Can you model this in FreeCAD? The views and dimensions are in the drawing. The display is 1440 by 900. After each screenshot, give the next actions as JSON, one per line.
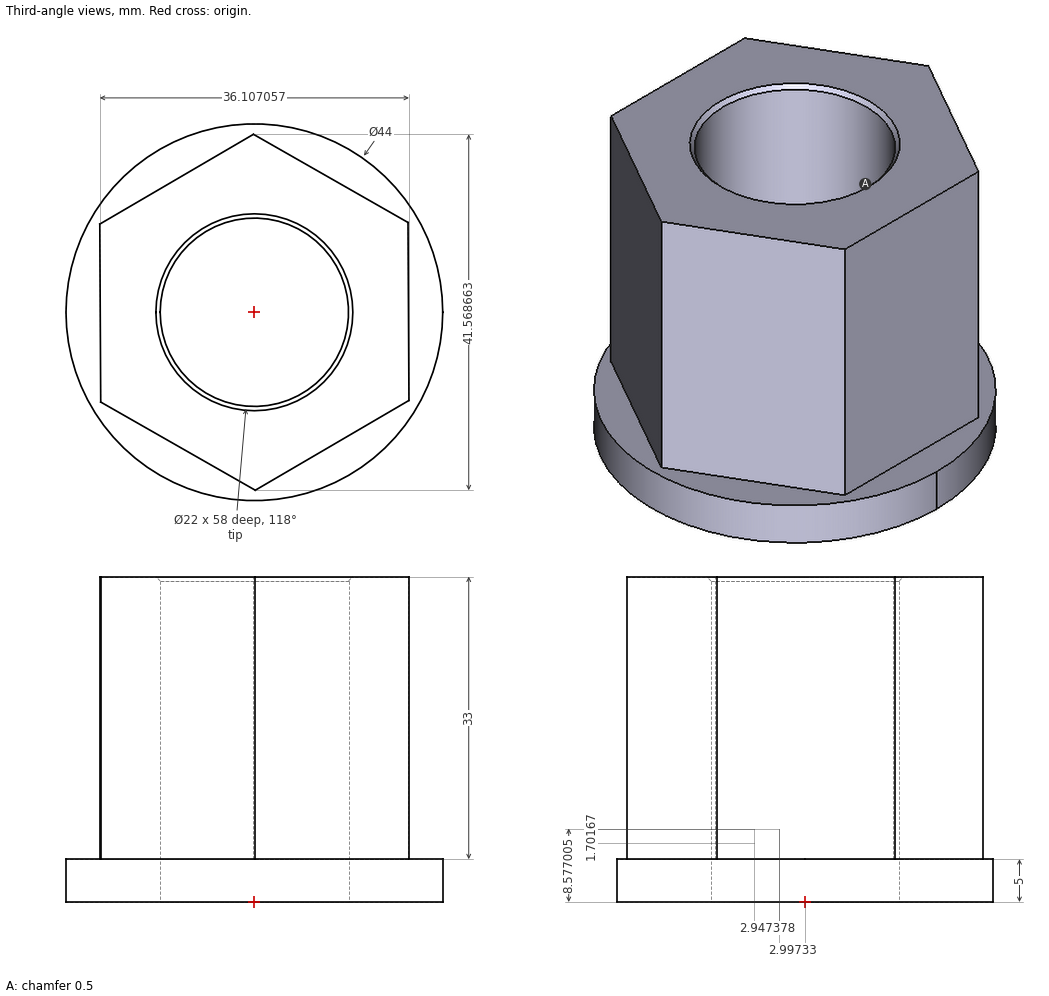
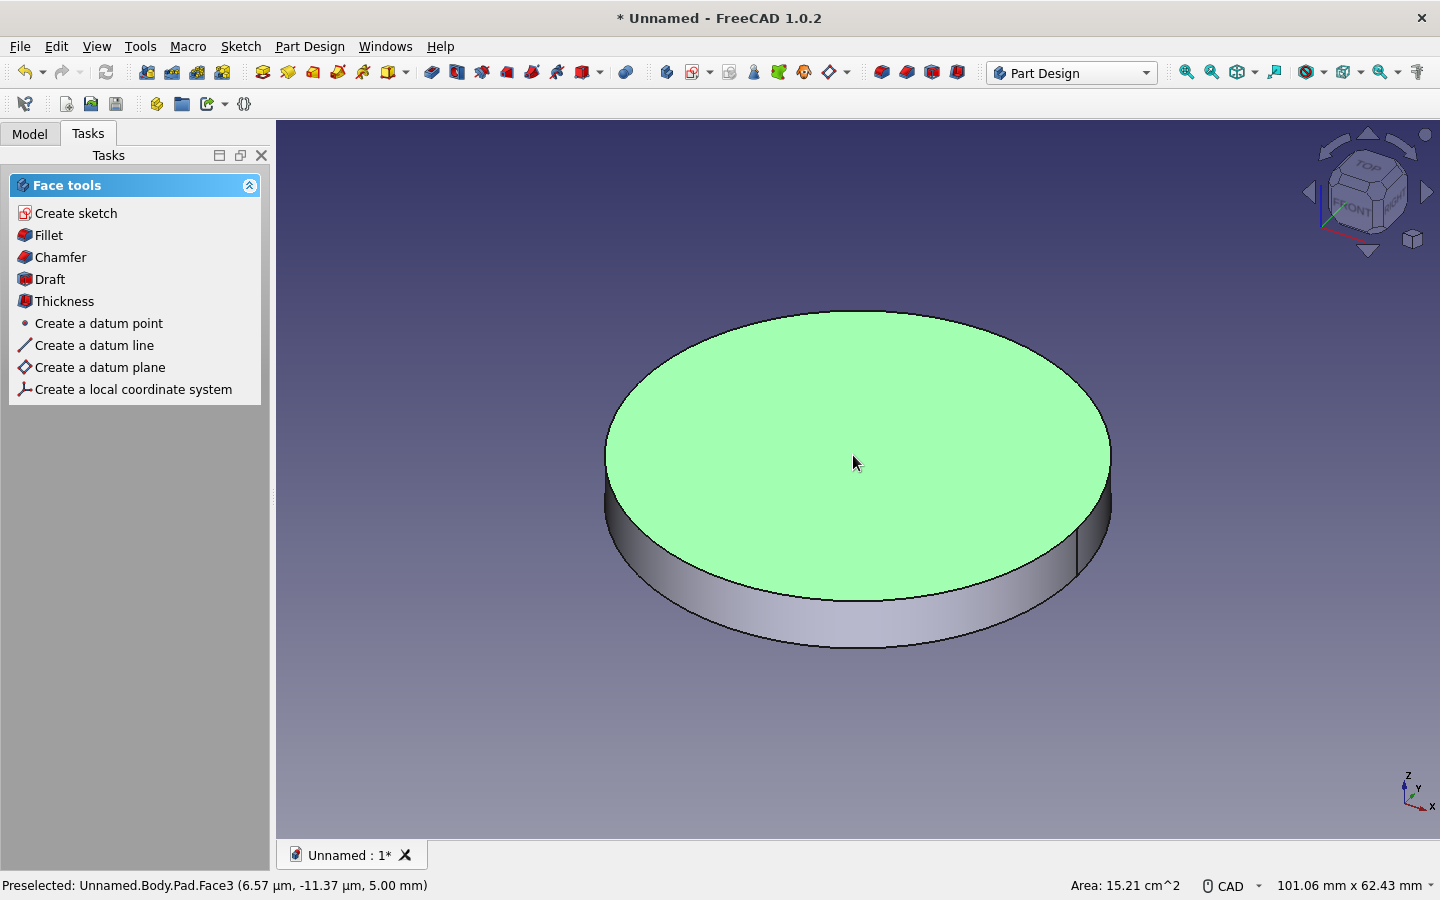
{"action": "left_click", "coordinate": [692, 72]}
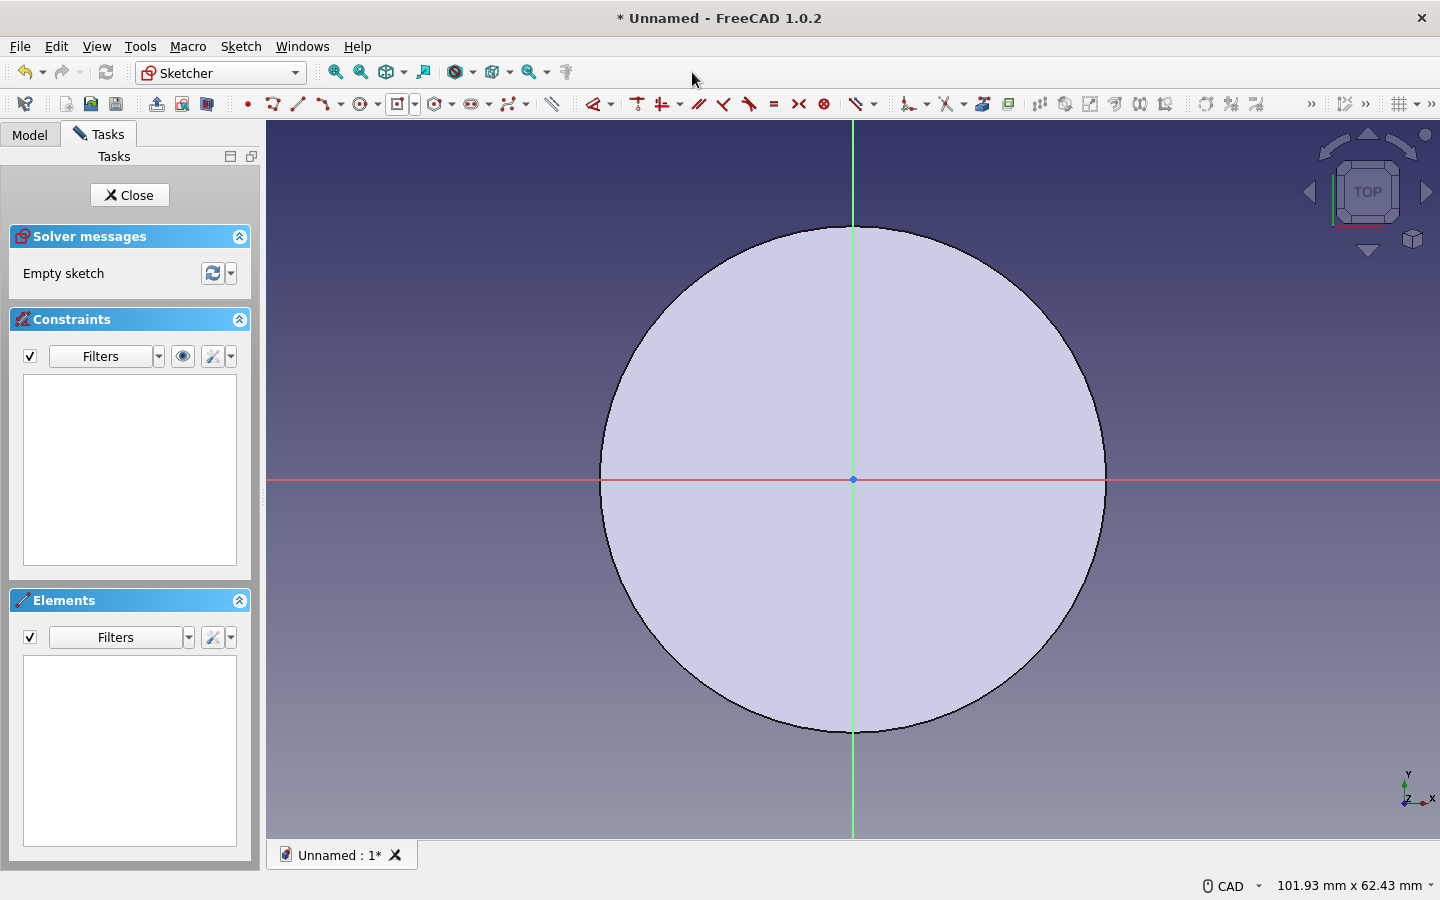
{"action": "key", "text": "g p 6"}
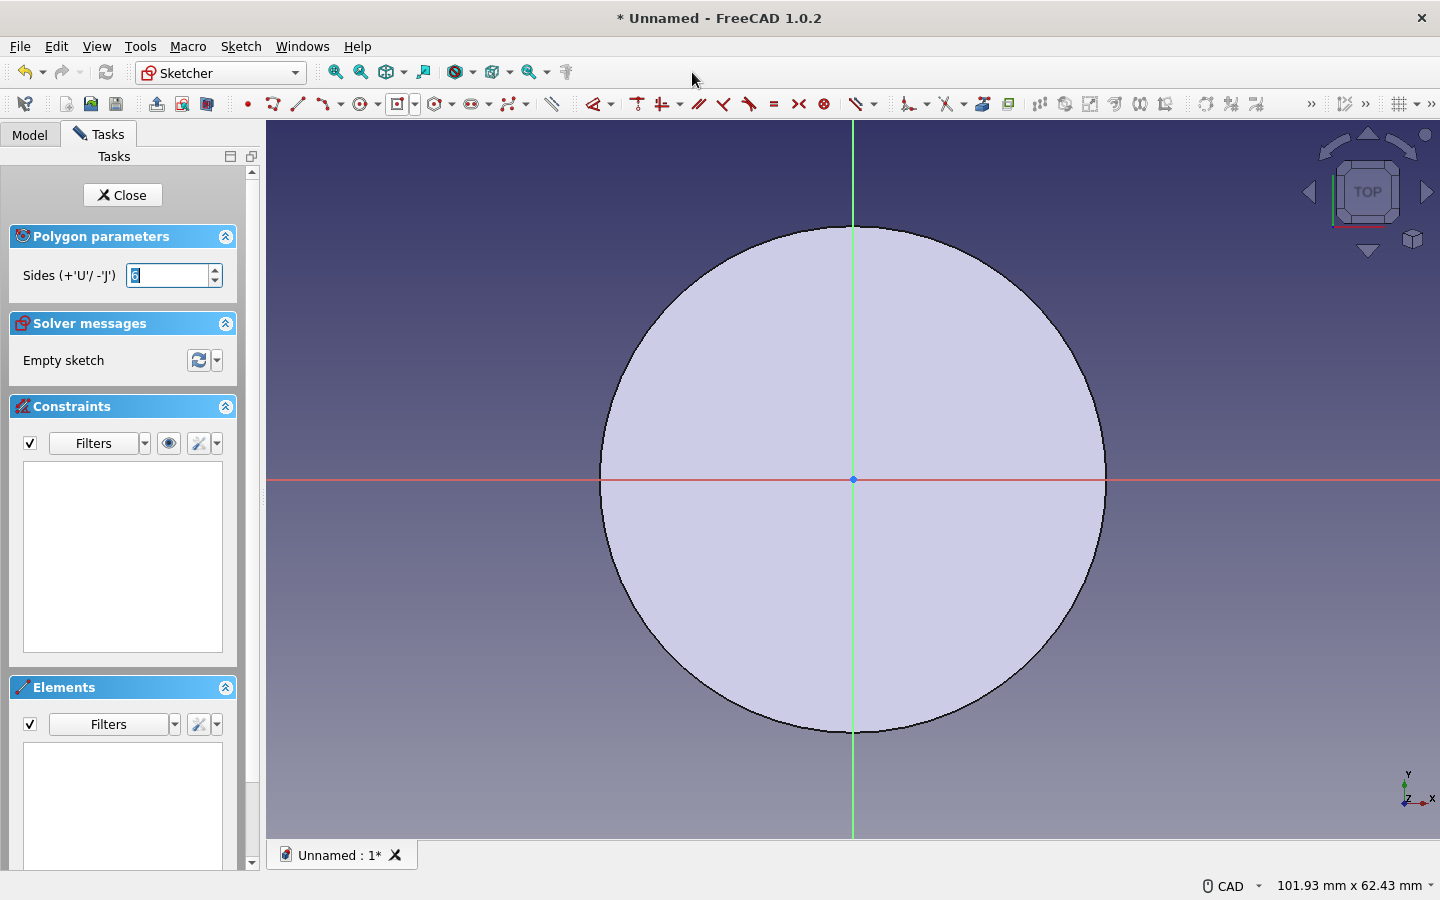
{"action": "left_click", "coordinate": [853, 480]}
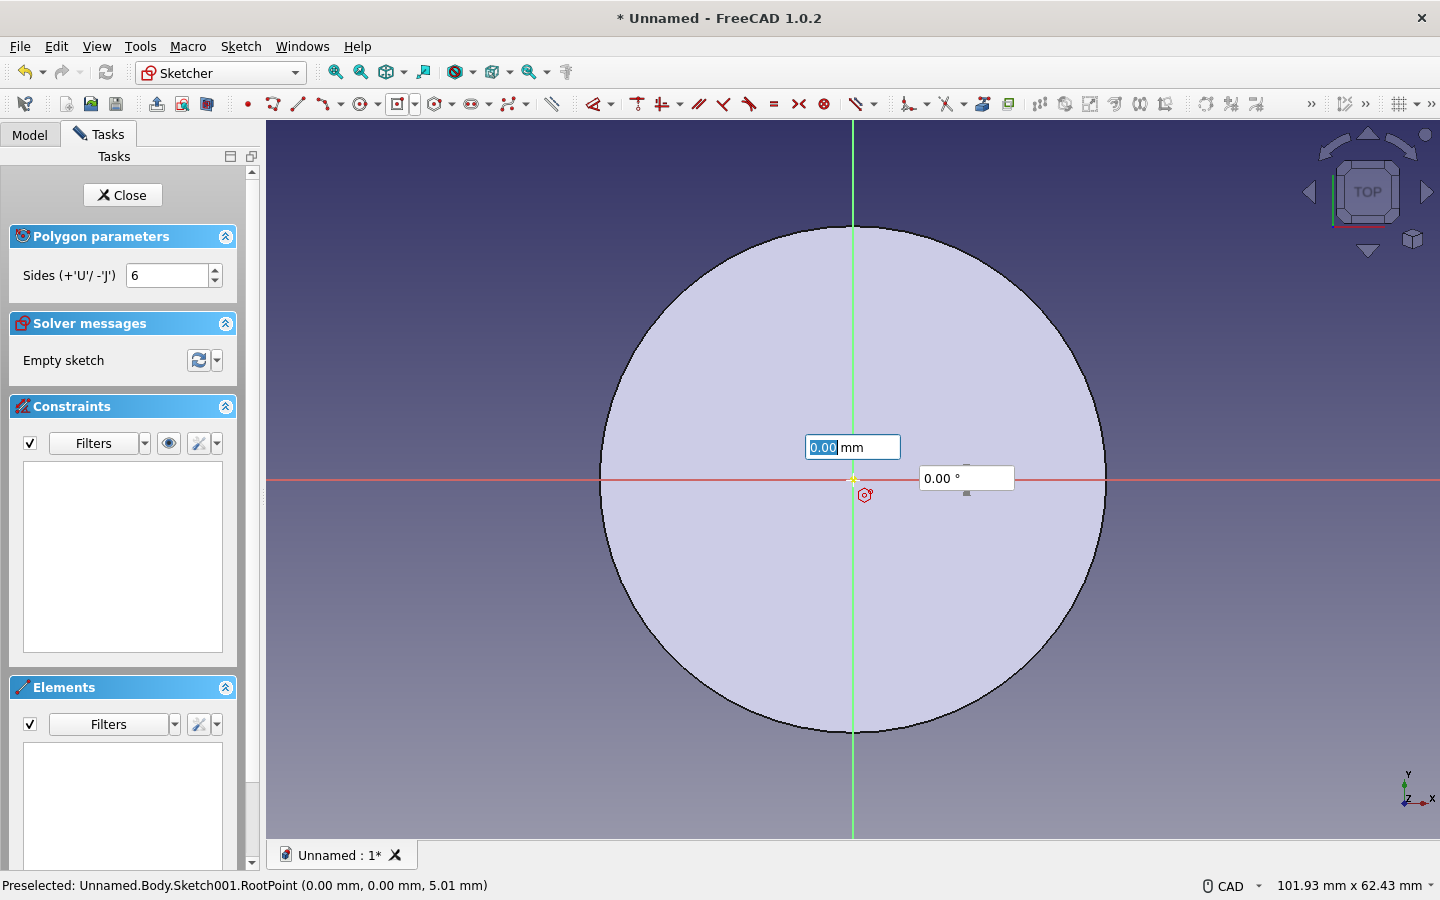
{"action": "left_click", "coordinate": [646, 600]}
{"action": "right_click", "coordinate": [646, 600]}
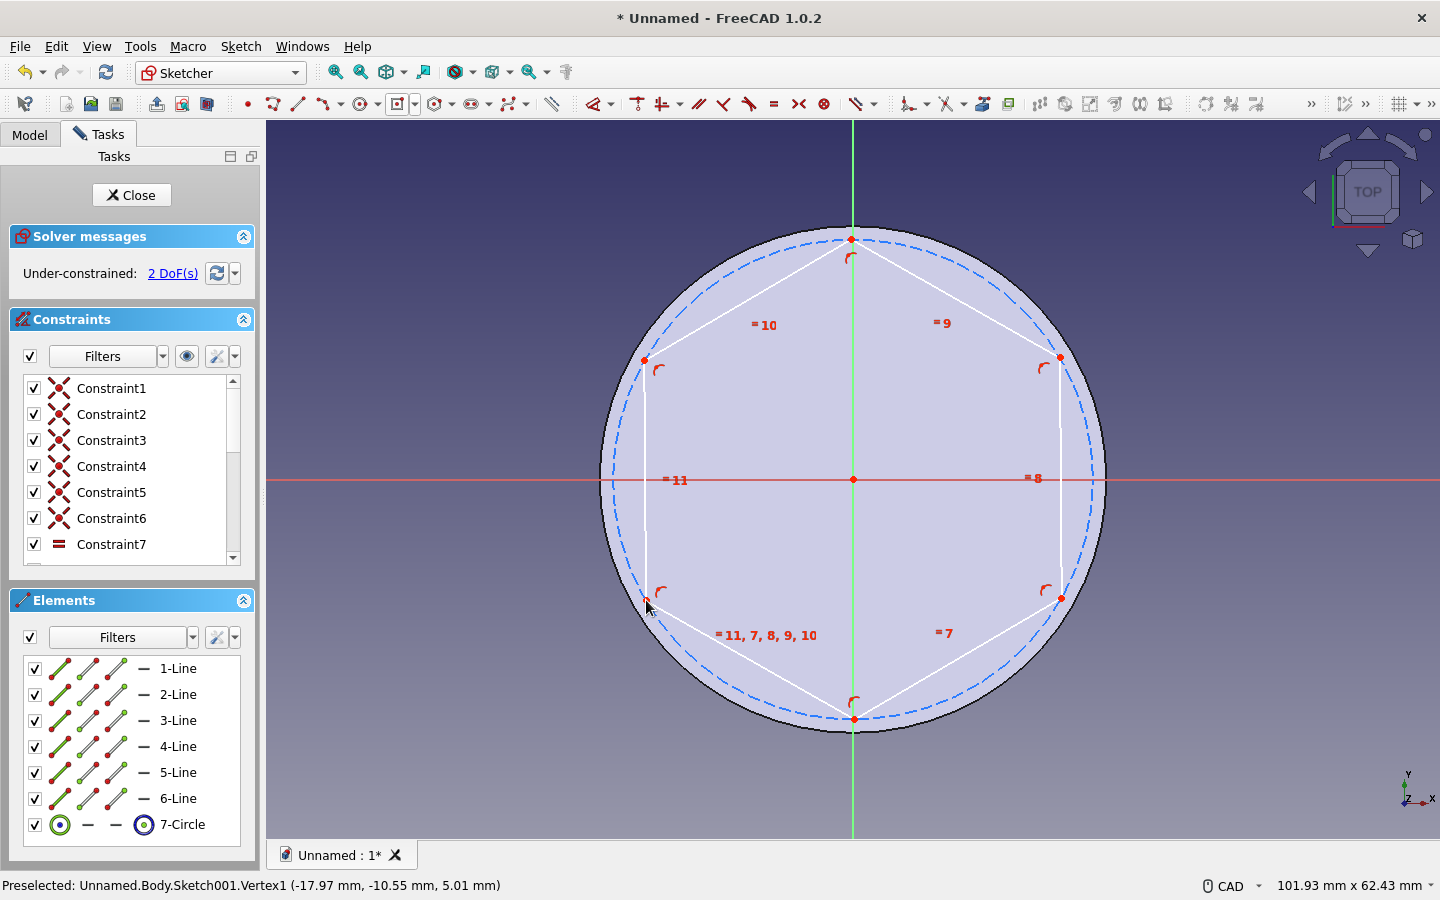
{"action": "left_click", "coordinate": [644, 361]}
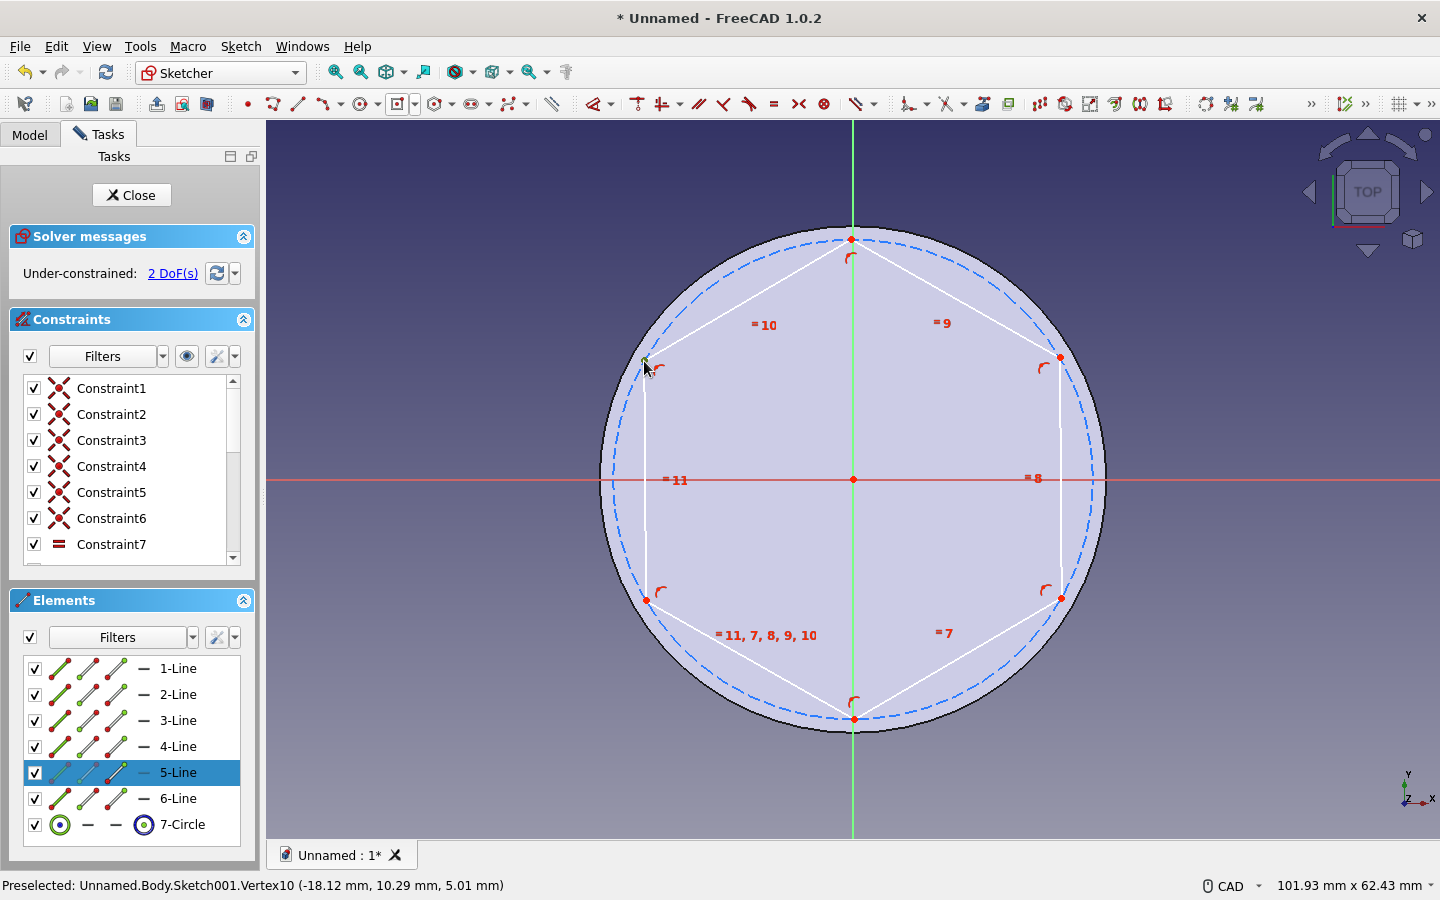
{"action": "left_click", "coordinate": [1062, 598]}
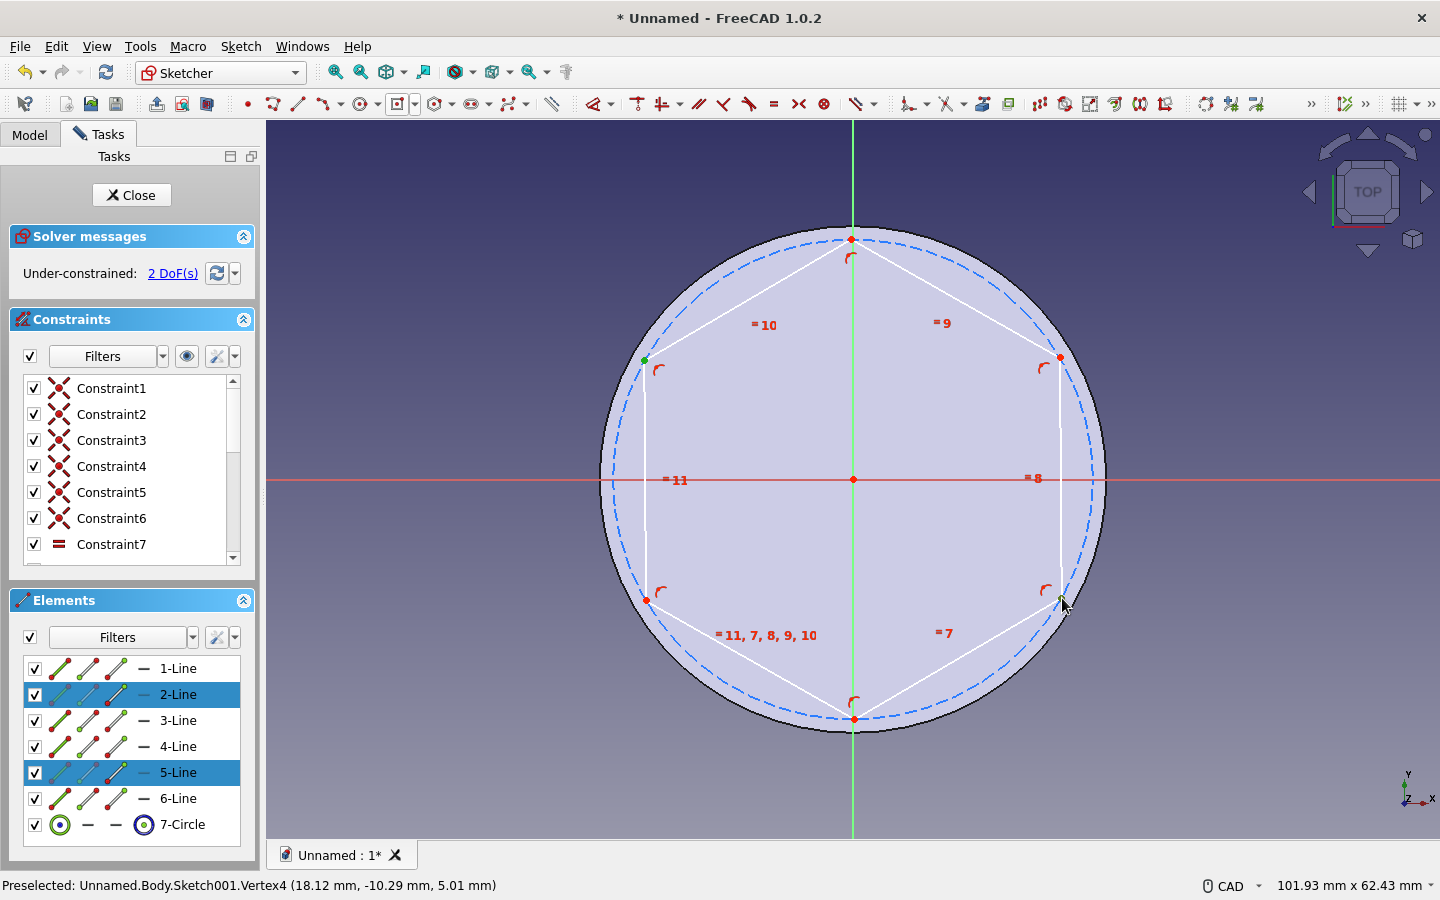
{"action": "key", "text": "l"}